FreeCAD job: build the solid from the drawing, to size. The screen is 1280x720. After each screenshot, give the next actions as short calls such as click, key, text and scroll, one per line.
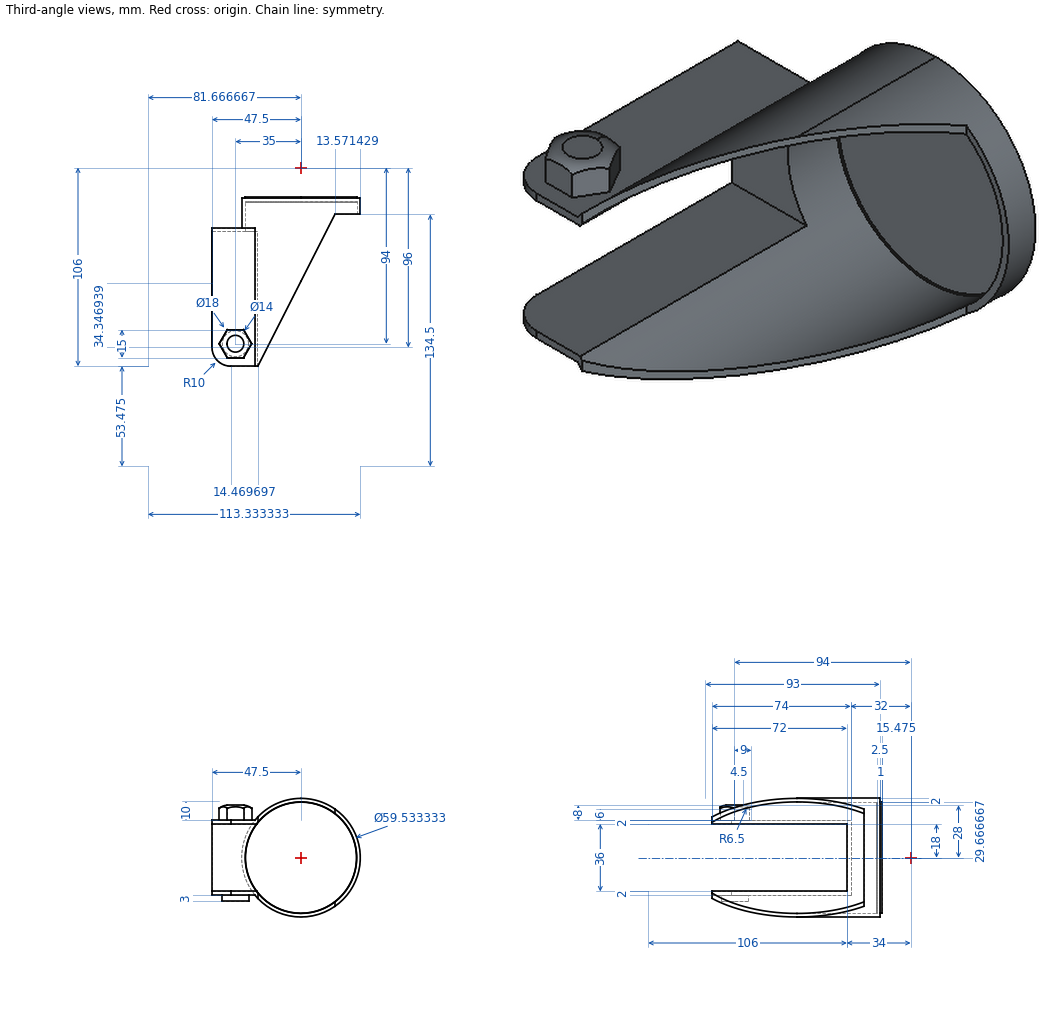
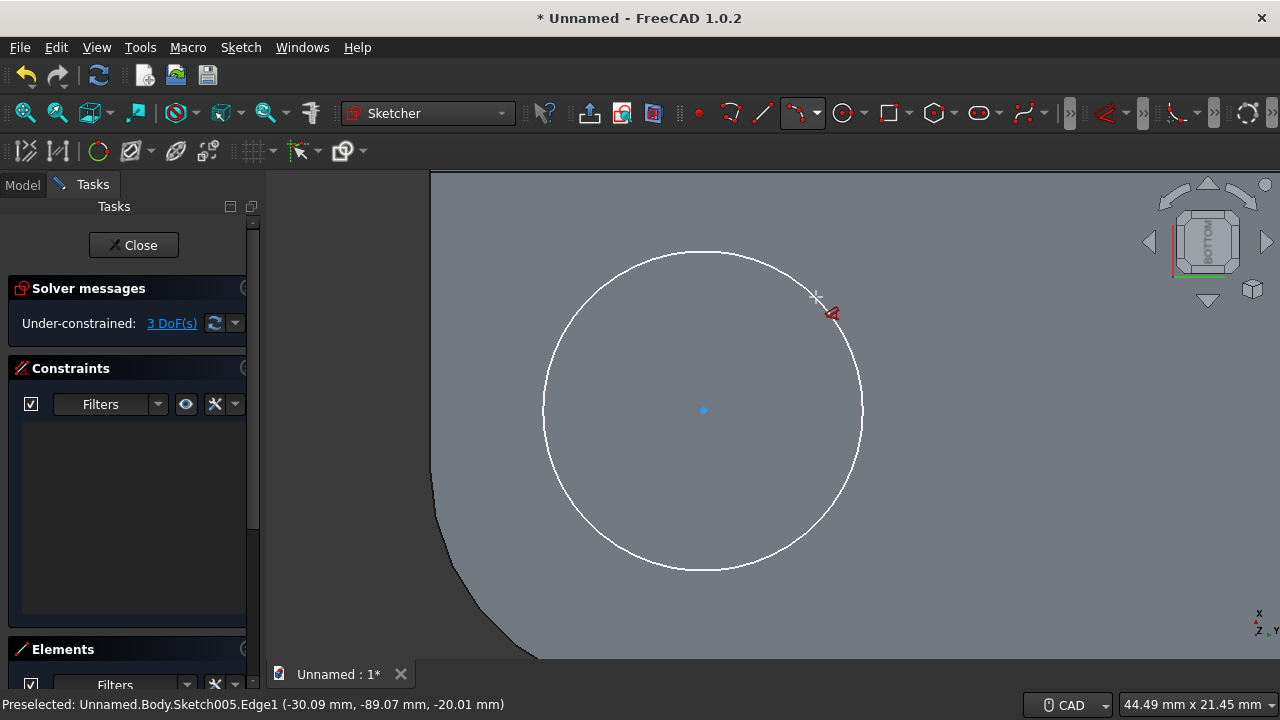
click(816, 298)
click(839, 275)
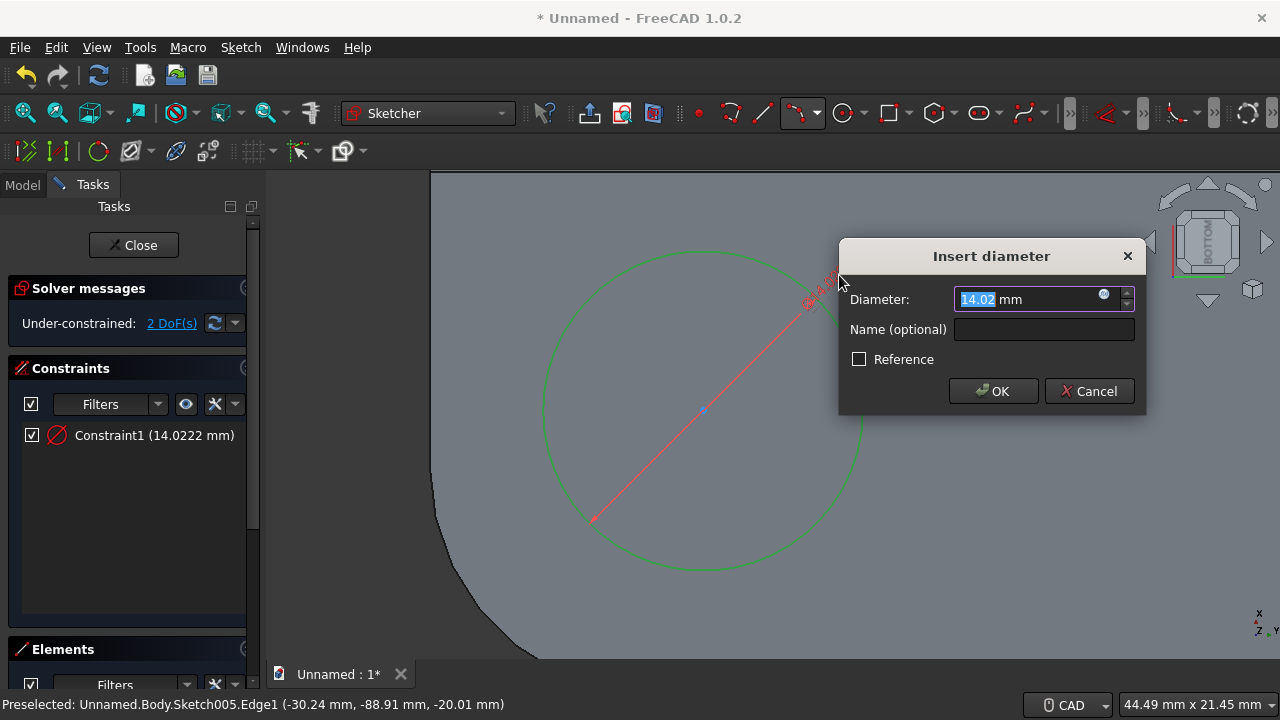
text(14)
key(Return)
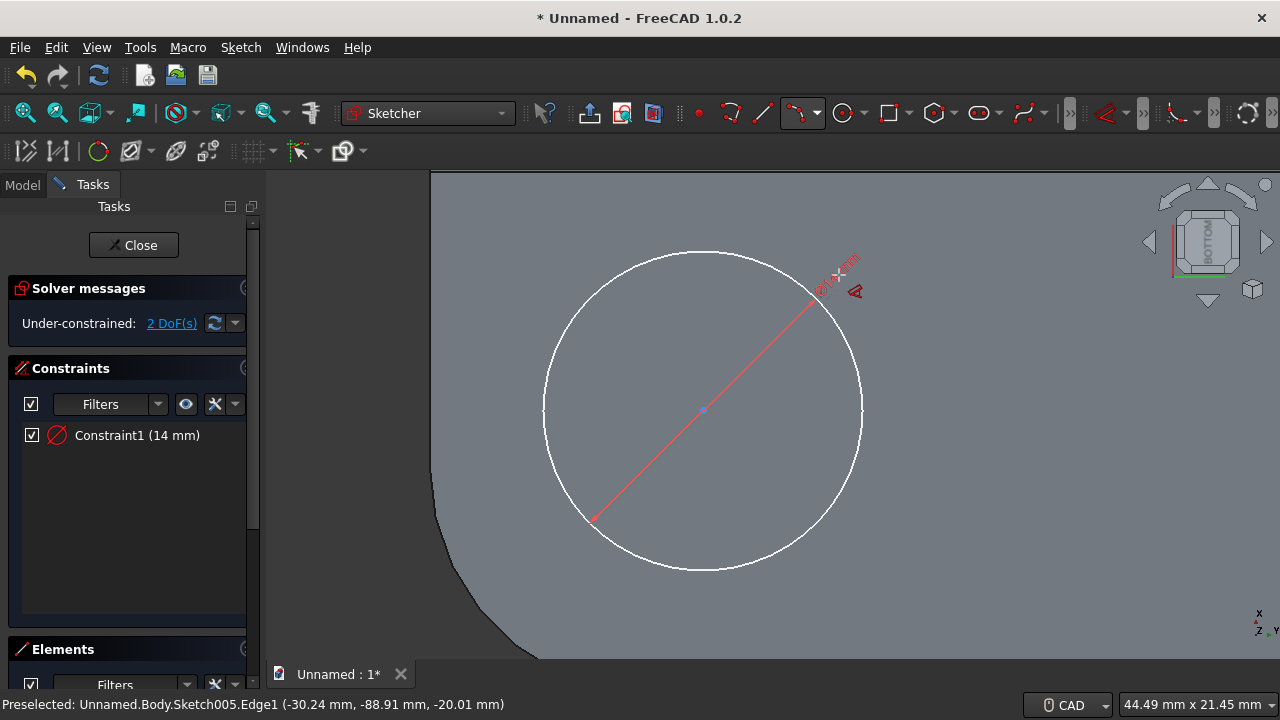
click(703, 411)
click(909, 445)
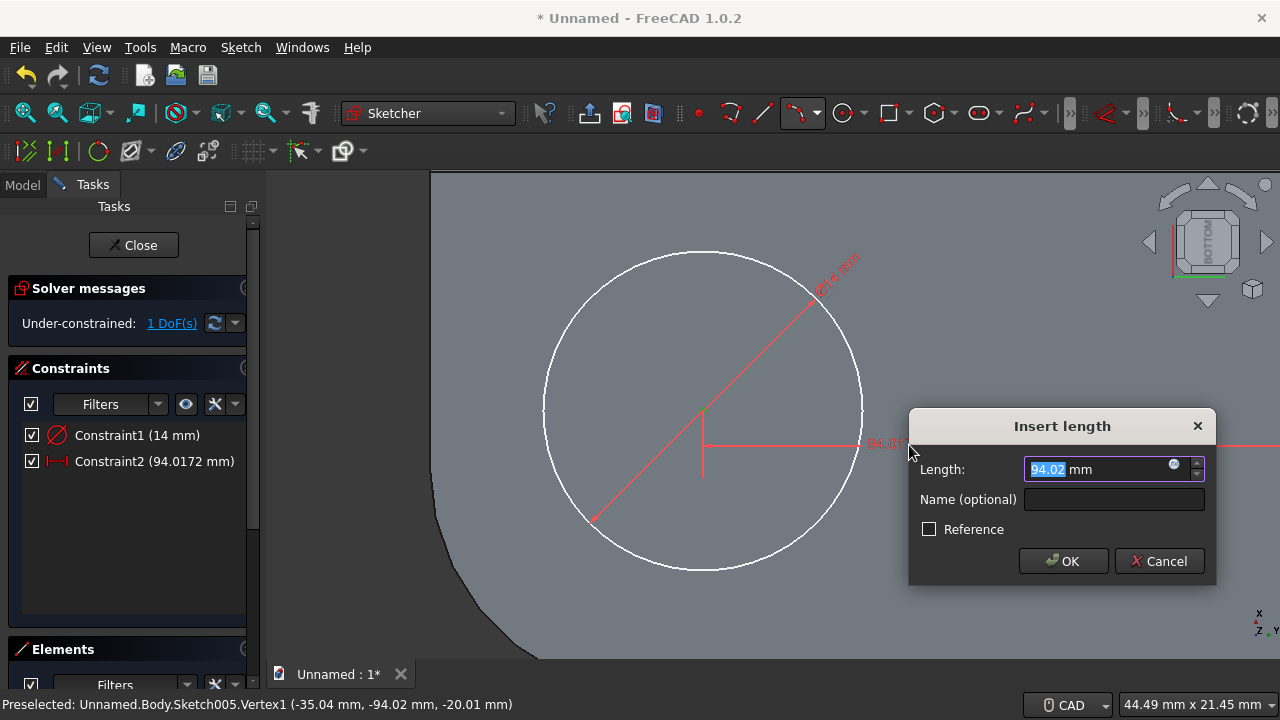
text(94)
key(Return)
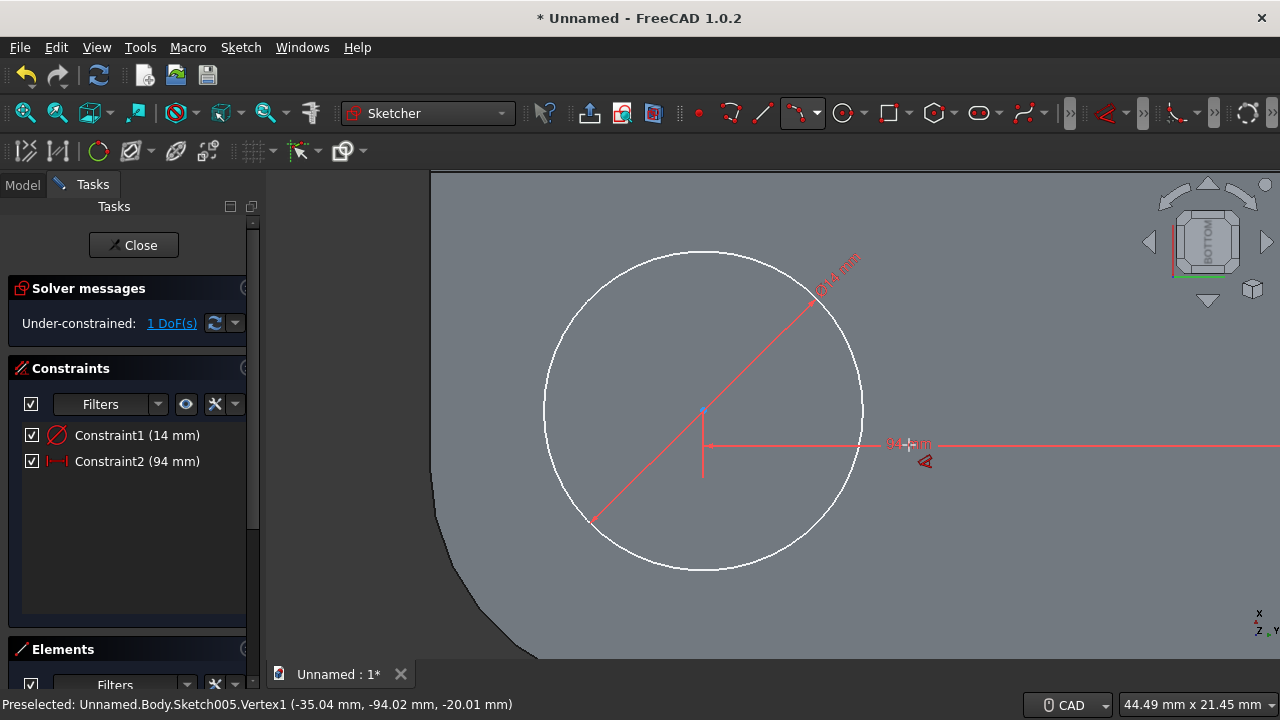
click(703, 411)
click(669, 305)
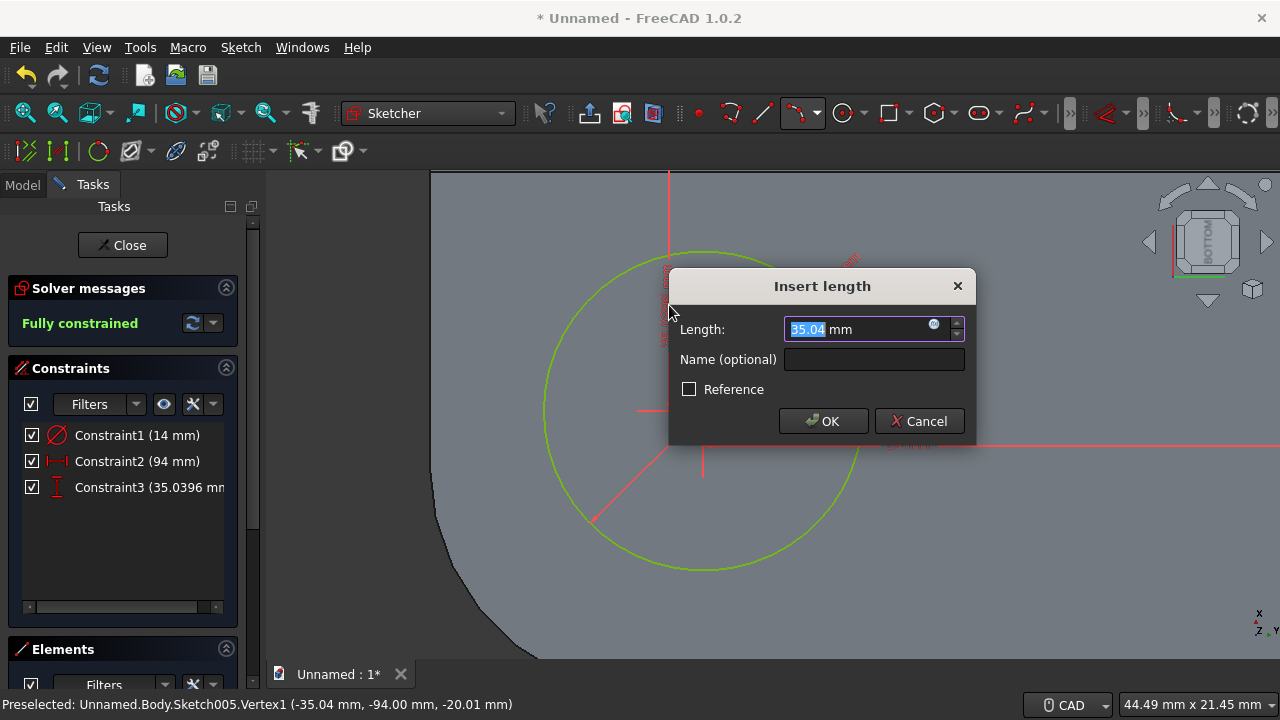
text(35)
key(Return)
key(Escape)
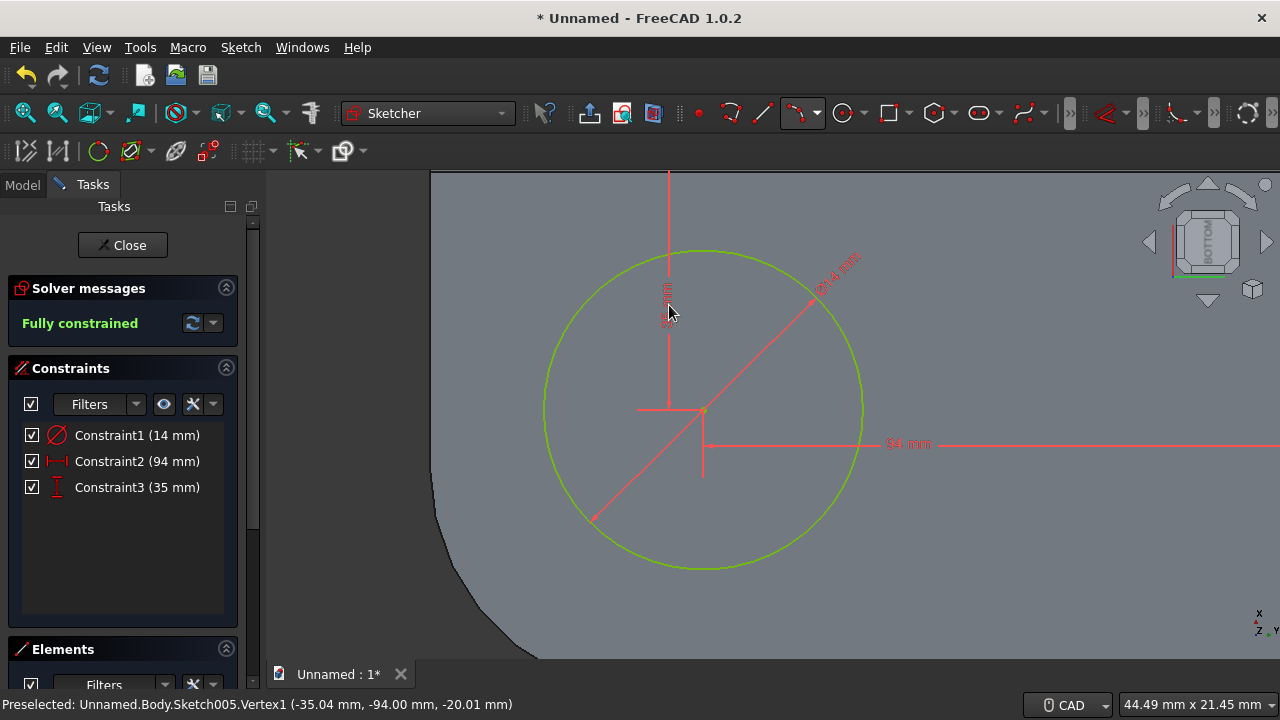
click(123, 245)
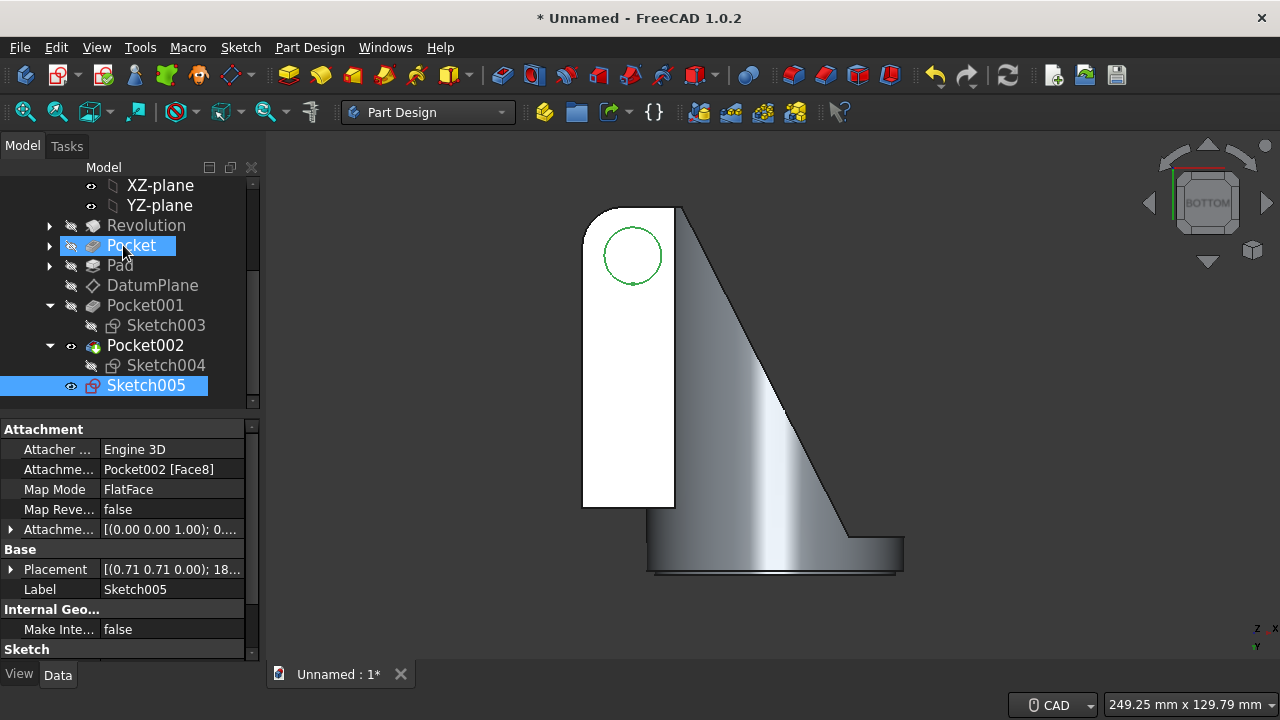
click(290, 76)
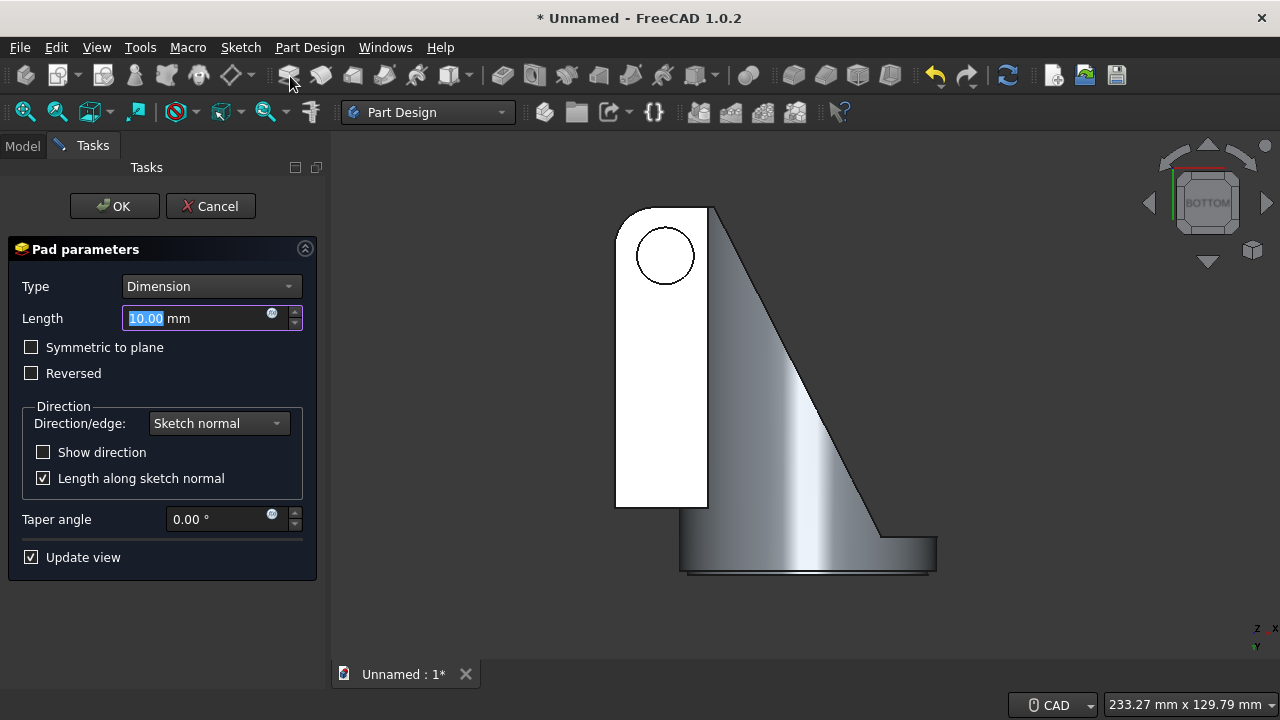
text(3)
key(Tab)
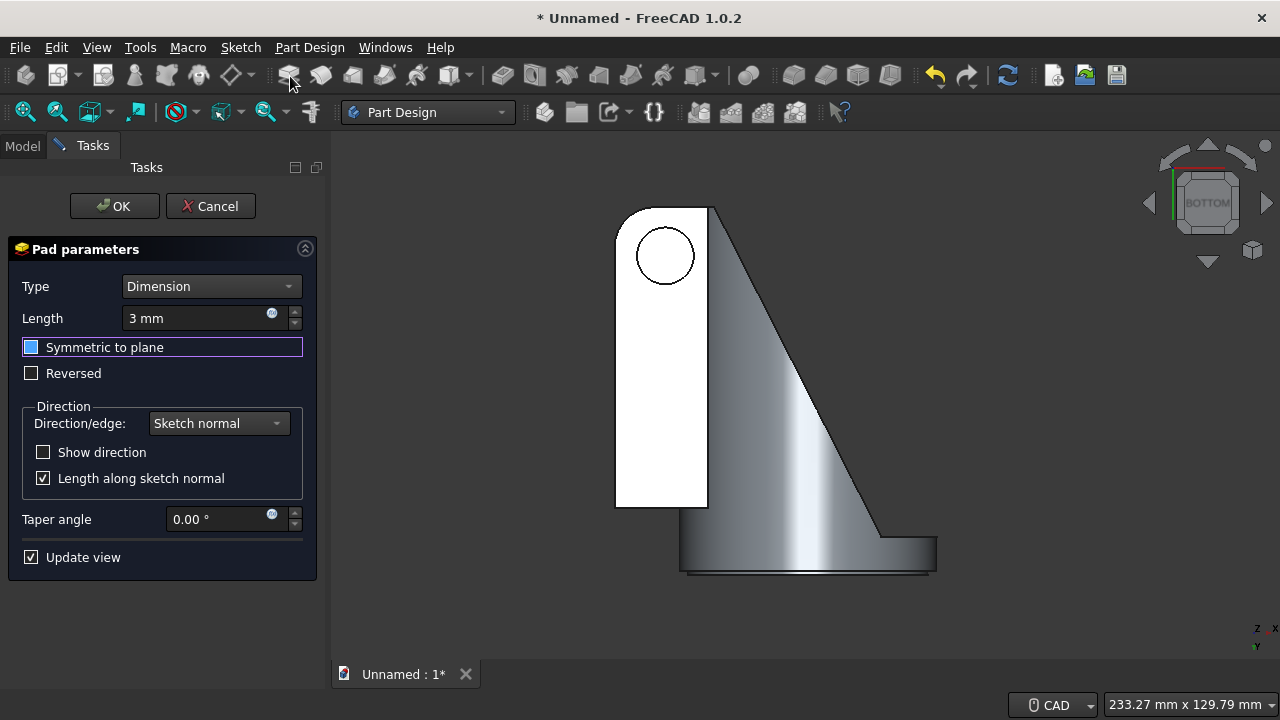
click(115, 206)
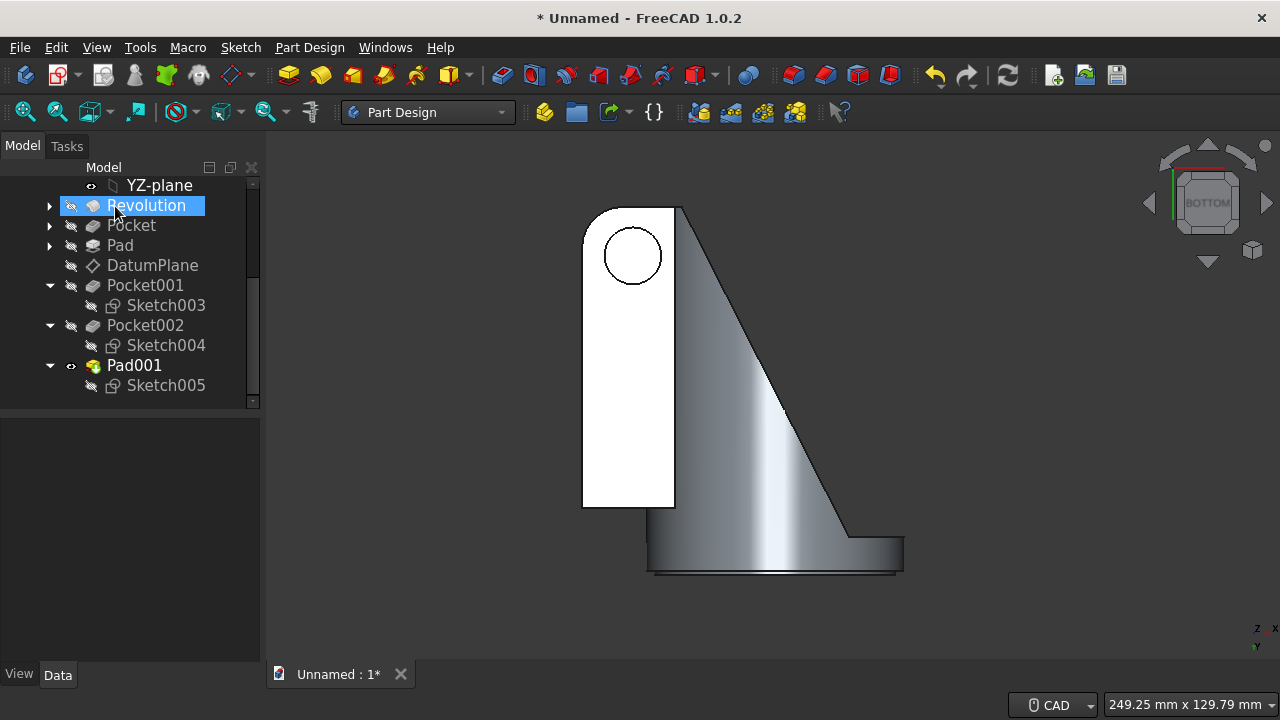
scroll(160, 281, down, 3)